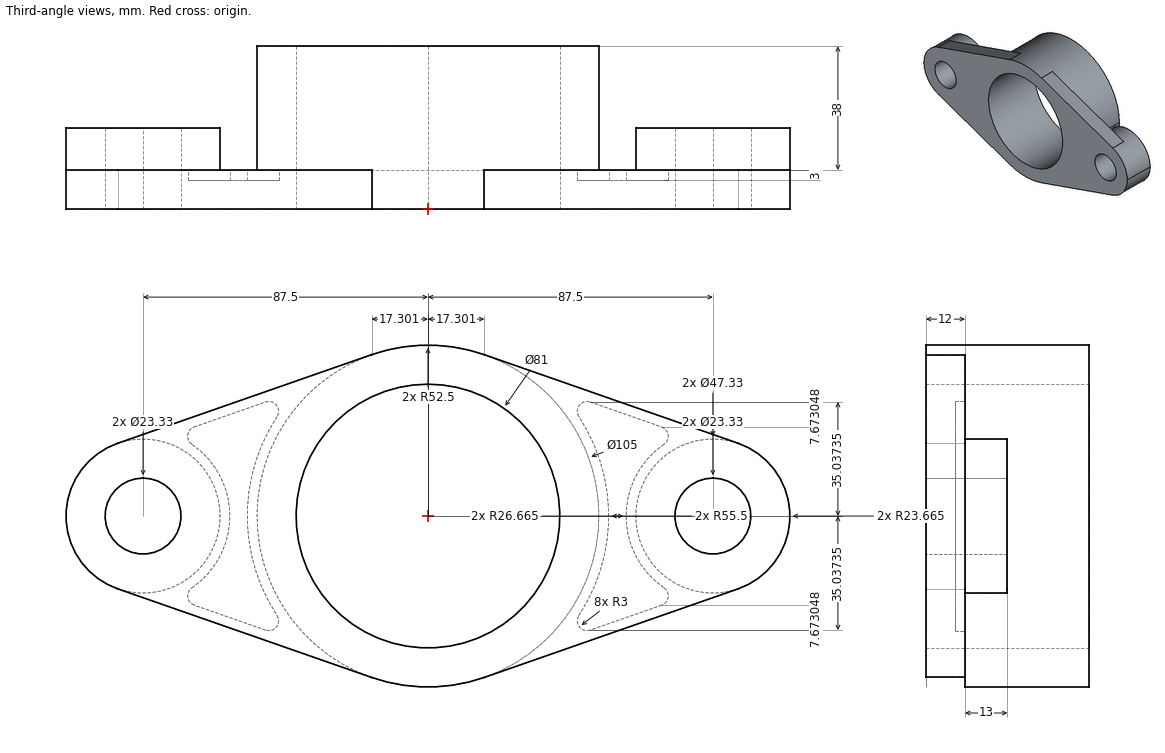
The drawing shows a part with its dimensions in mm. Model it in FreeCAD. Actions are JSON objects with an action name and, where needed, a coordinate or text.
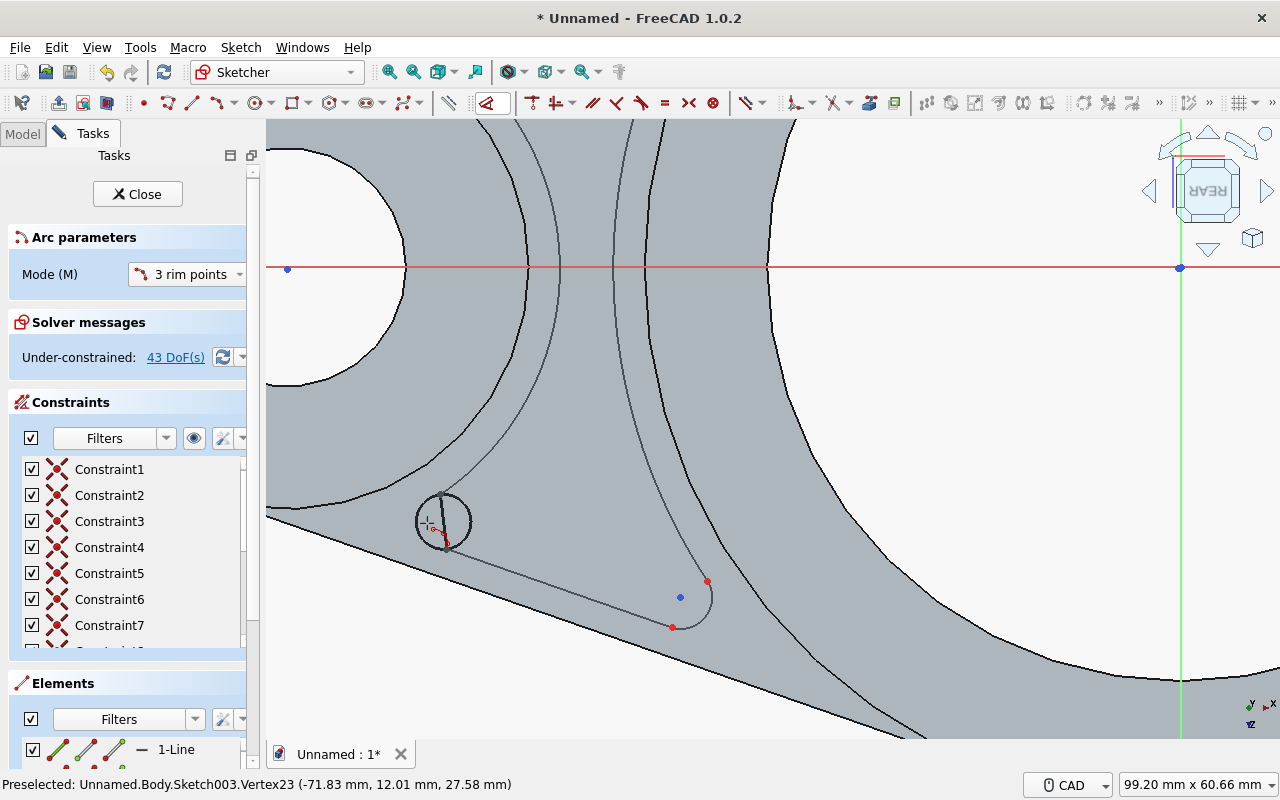
{"action": "left_click", "coordinate": [427, 522]}
{"action": "key", "text": "Escape"}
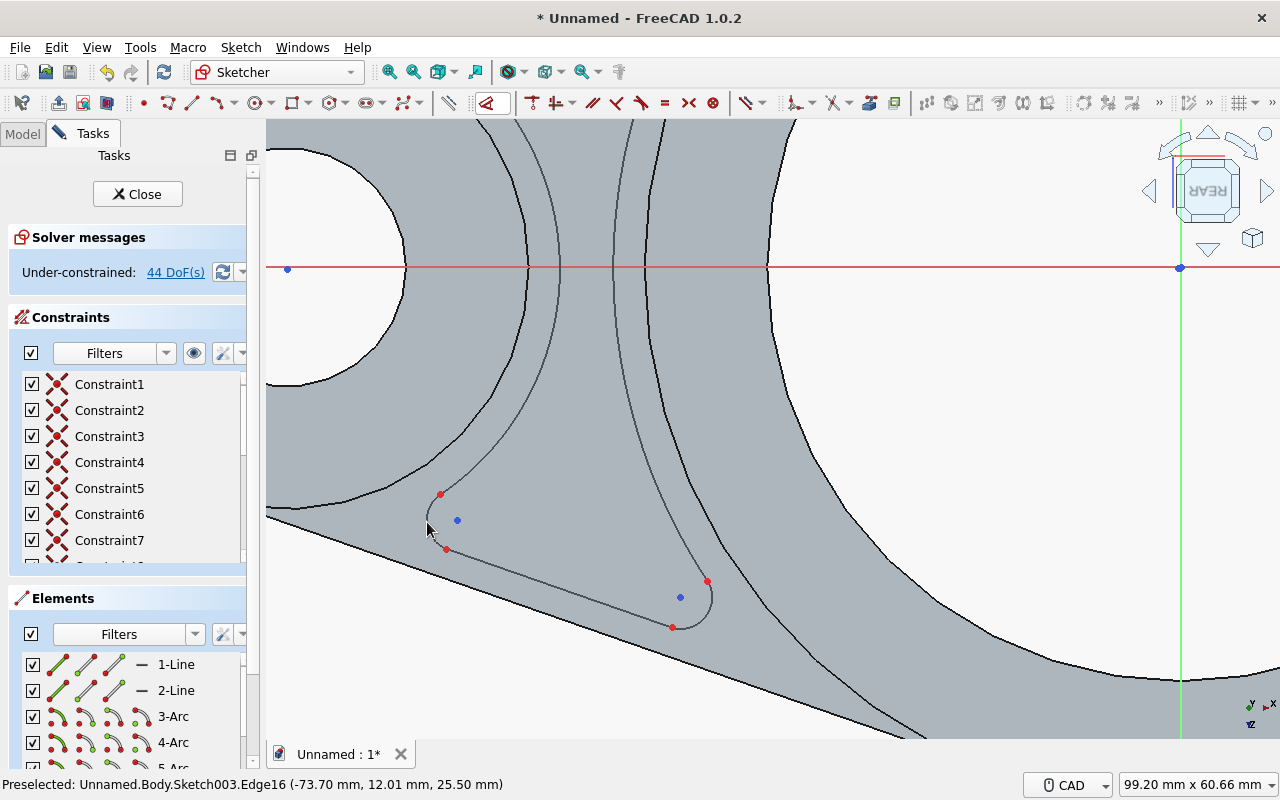
{"action": "scroll", "coordinate": [427, 523], "scroll_direction": "down", "scroll_amount": 5}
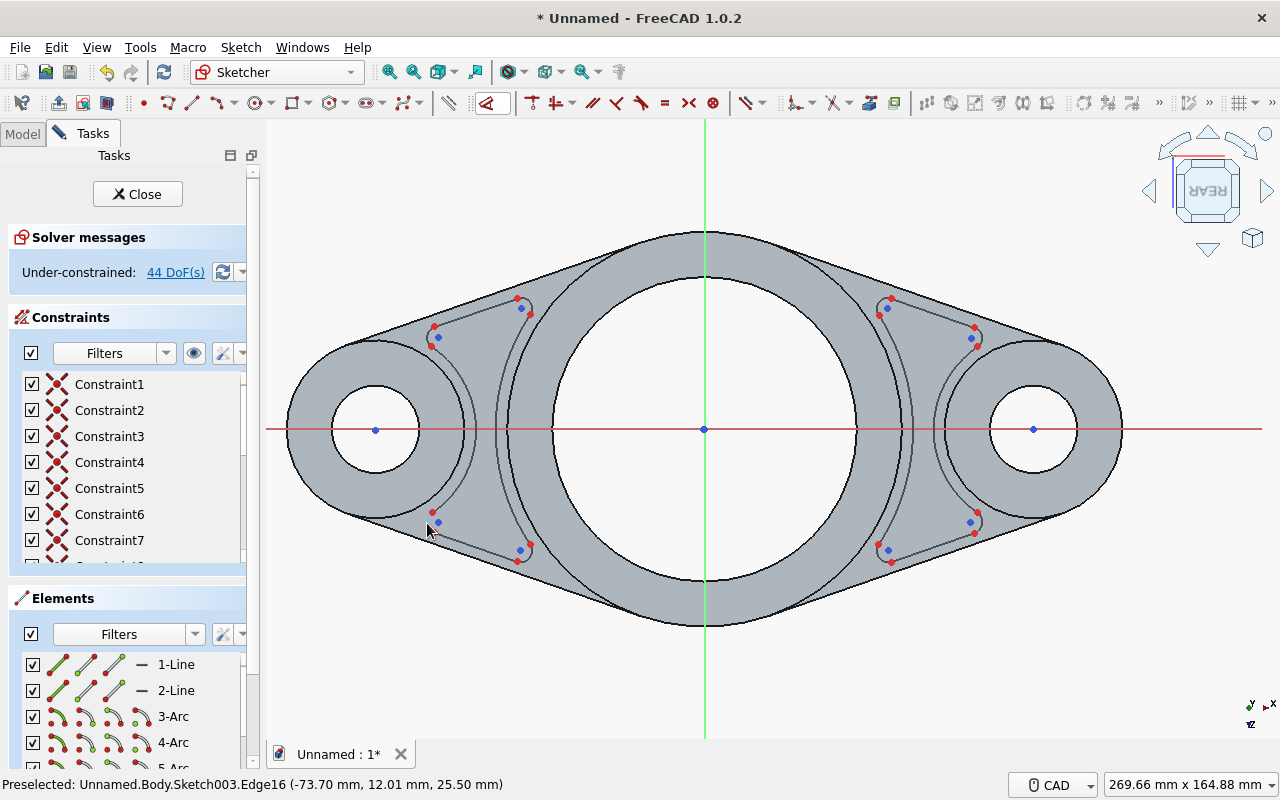
{"action": "left_click", "coordinate": [950, 319]}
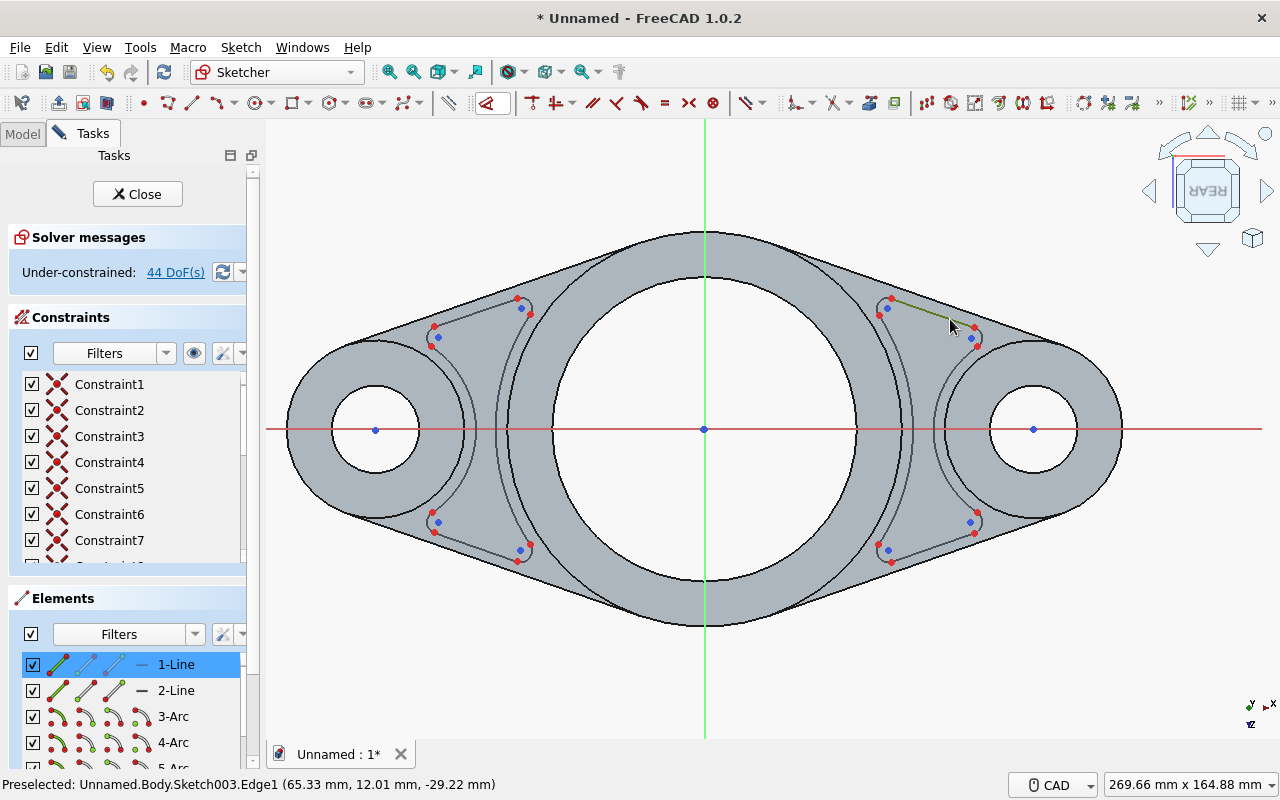
{"action": "scroll", "coordinate": [879, 302], "scroll_direction": "up", "scroll_amount": 2}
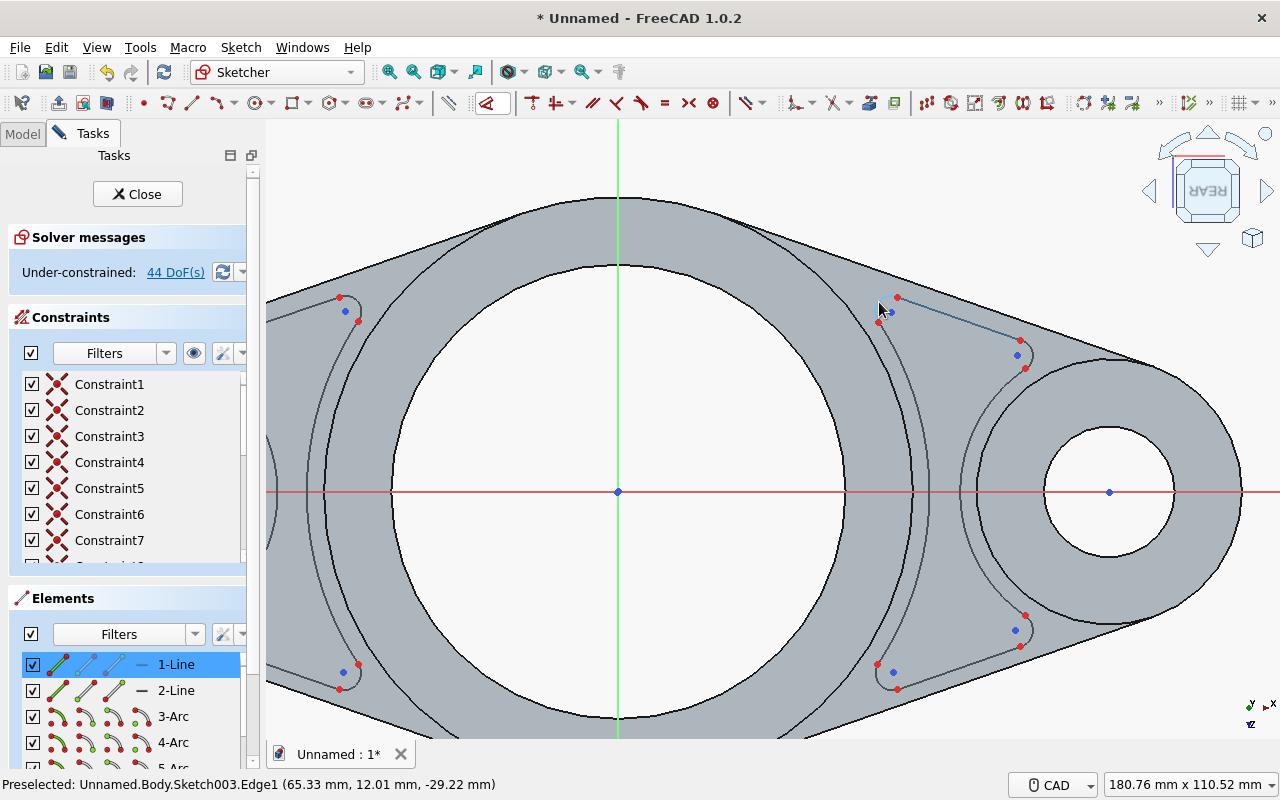
{"action": "left_click", "coordinate": [878, 302]}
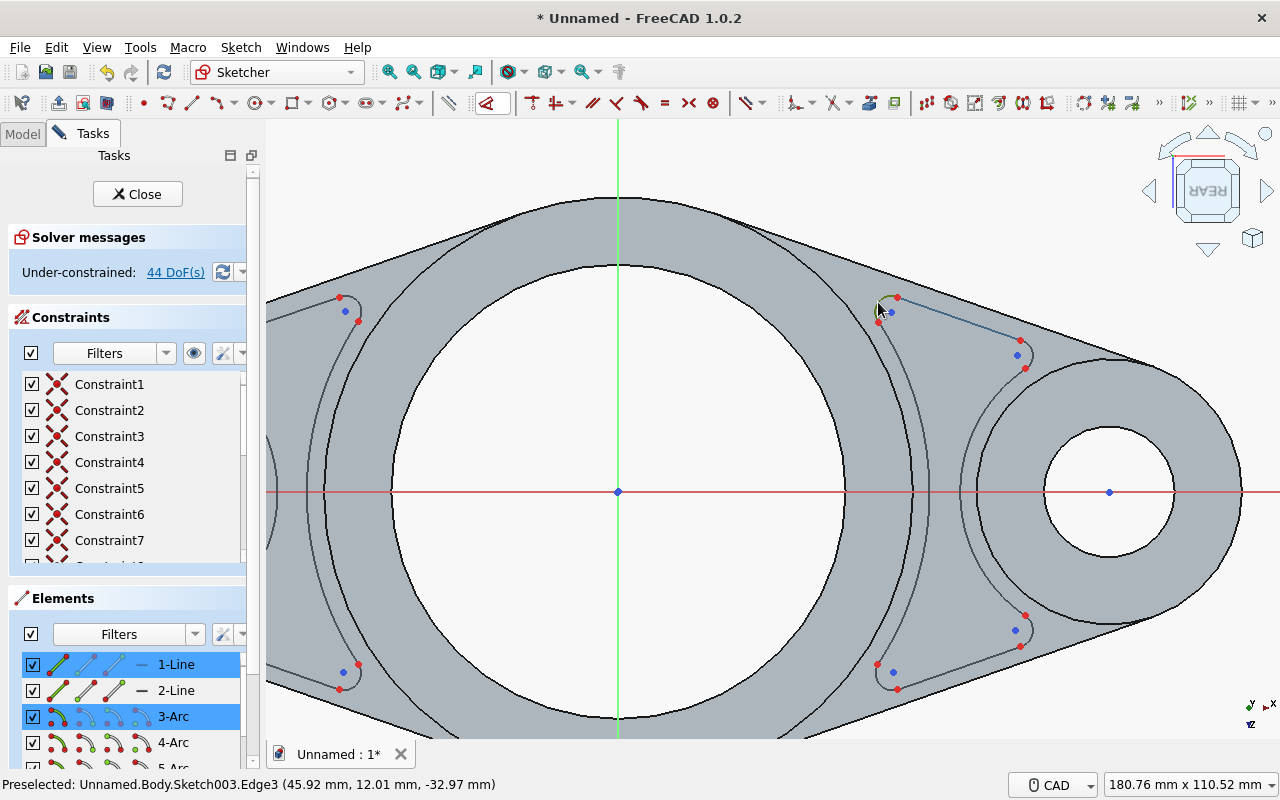
{"action": "left_click", "coordinate": [642, 104]}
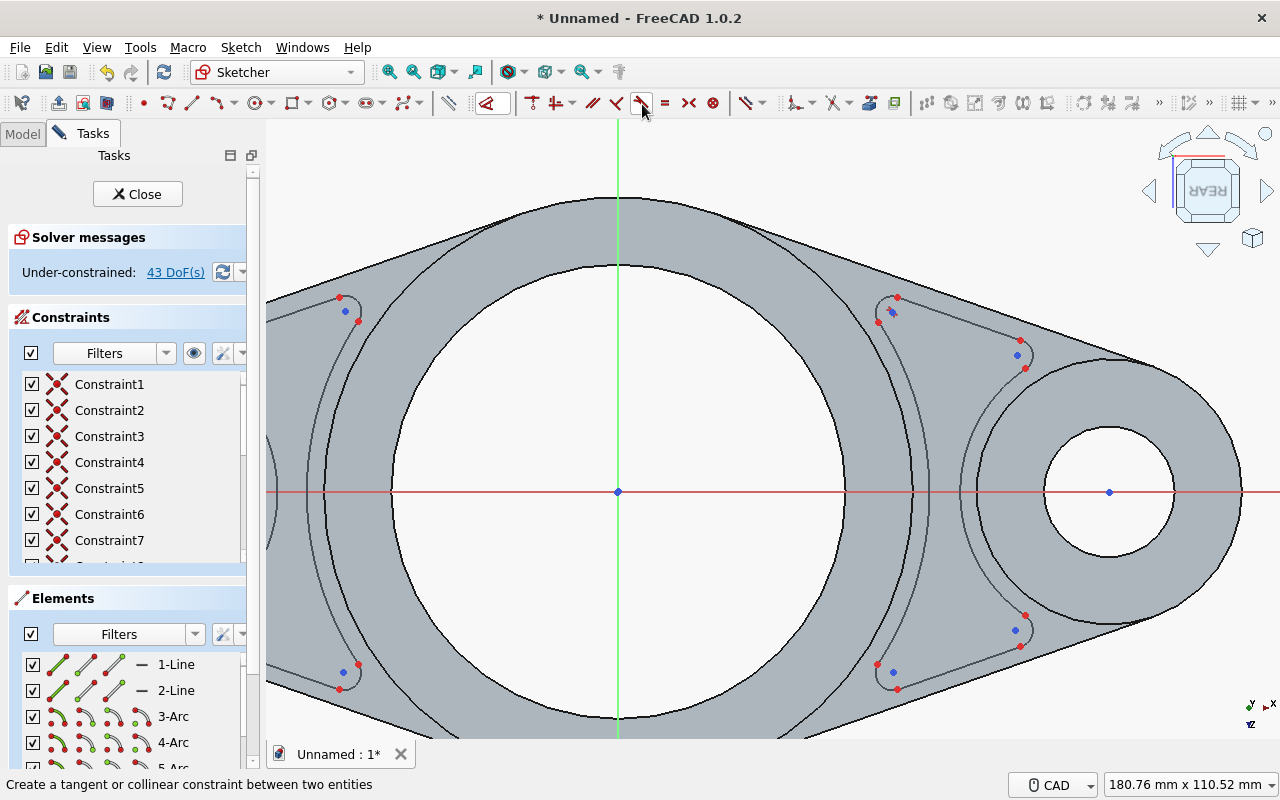
{"action": "left_click", "coordinate": [984, 328]}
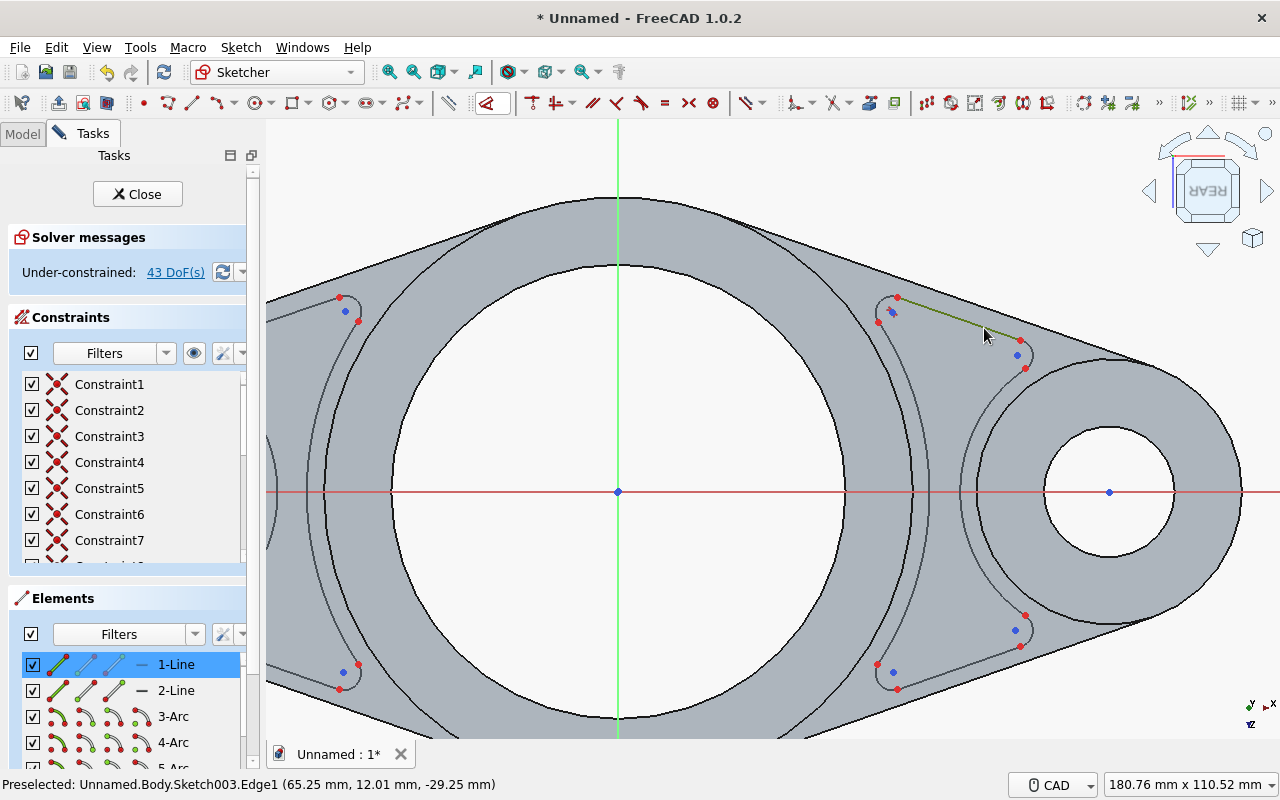
{"action": "scroll", "coordinate": [1032, 360], "scroll_direction": "up", "scroll_amount": 2}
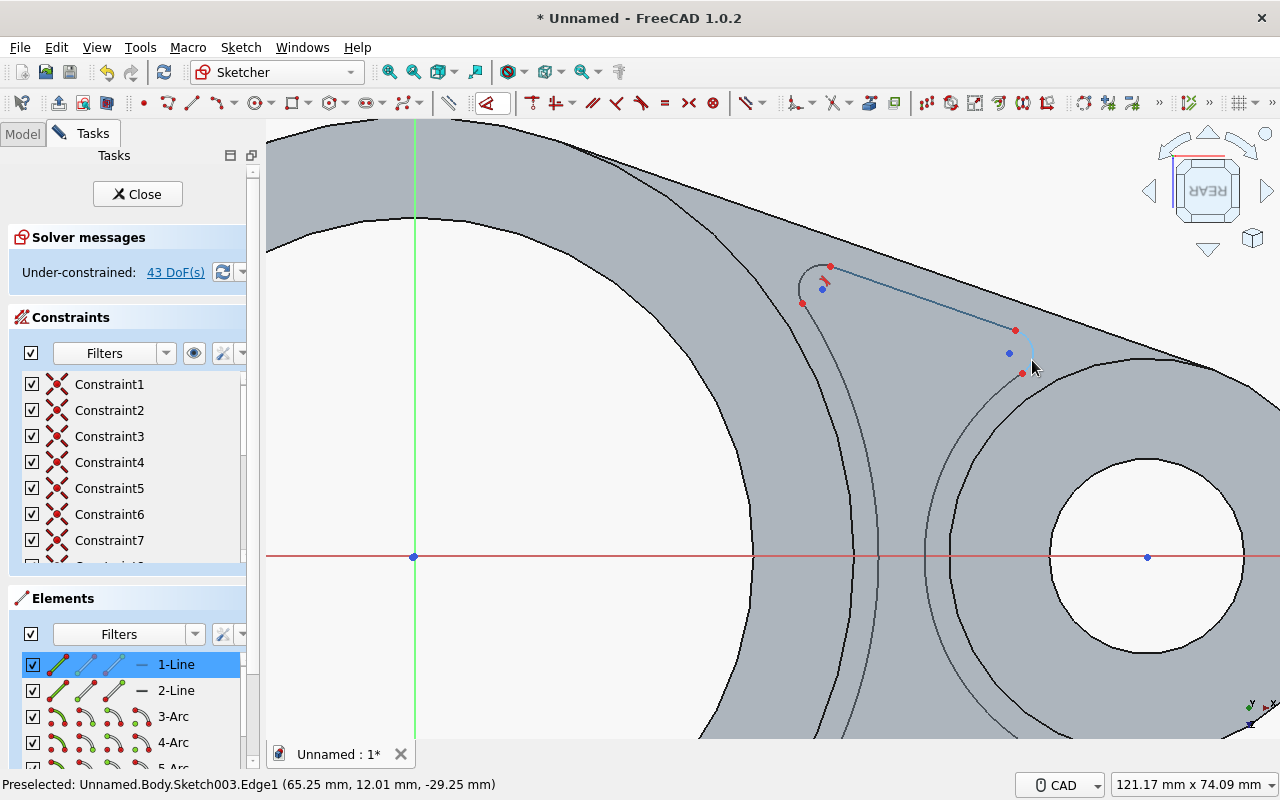
{"action": "left_click", "coordinate": [1032, 360]}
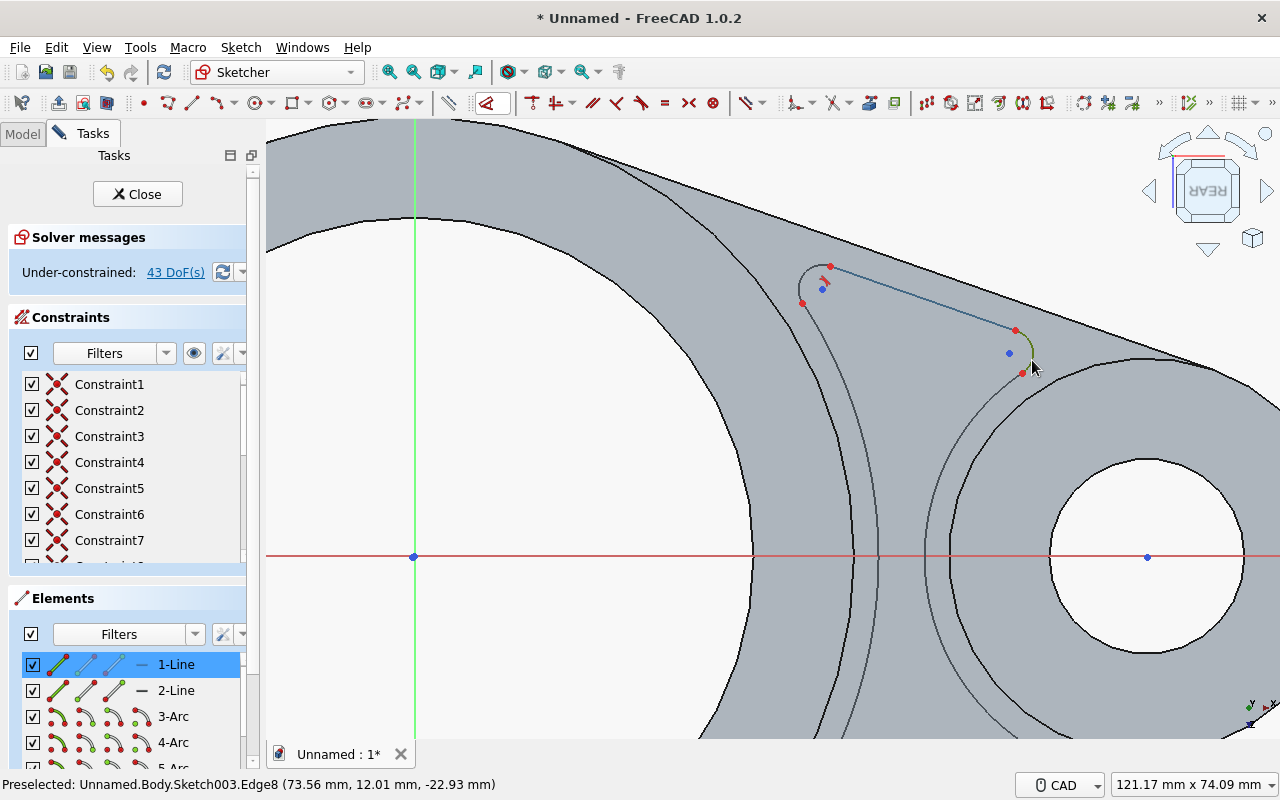
{"action": "left_click", "coordinate": [642, 104]}